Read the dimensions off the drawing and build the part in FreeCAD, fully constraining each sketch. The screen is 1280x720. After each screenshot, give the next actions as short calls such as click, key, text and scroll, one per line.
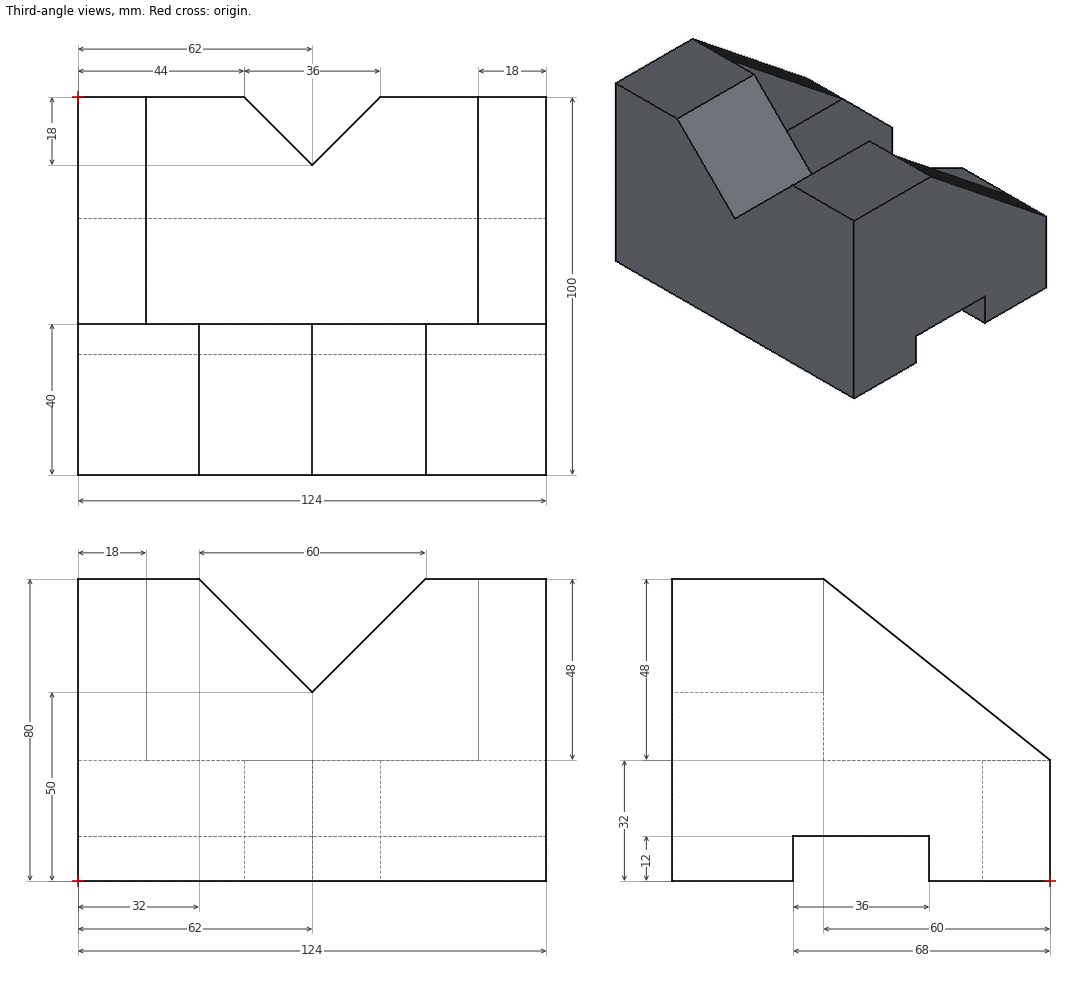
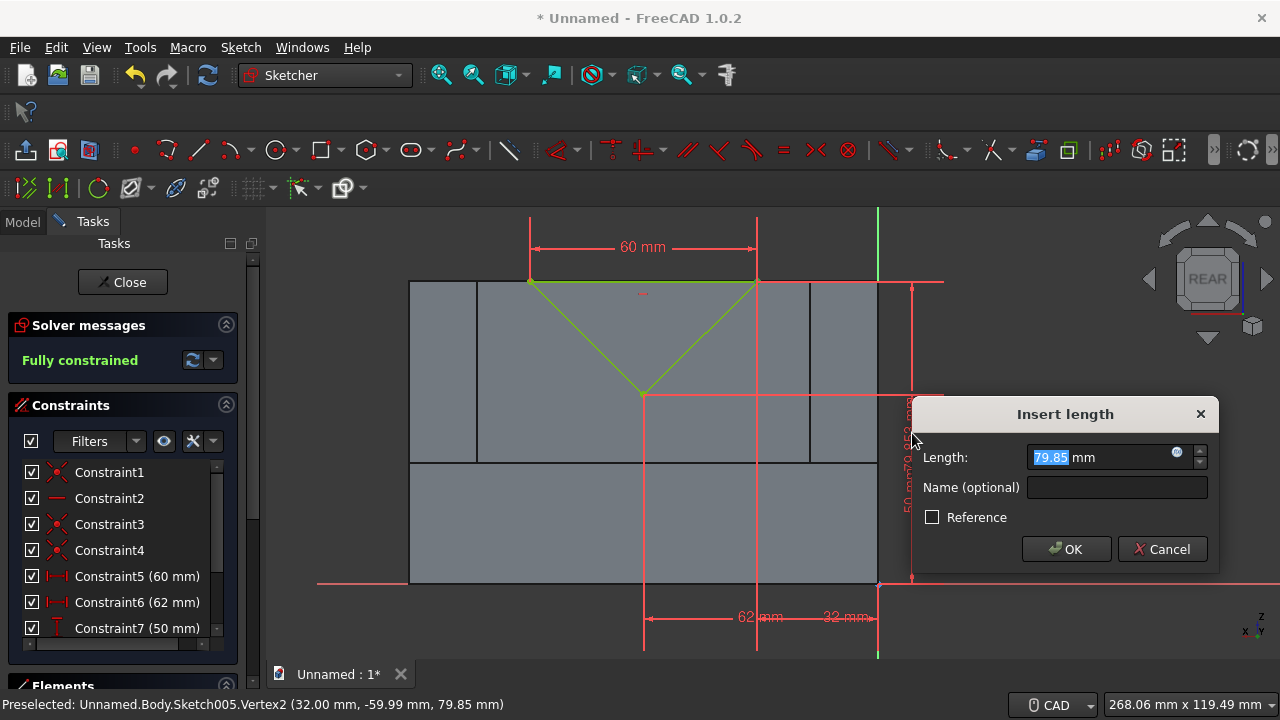
text(80)
key(Return)
key(Escape)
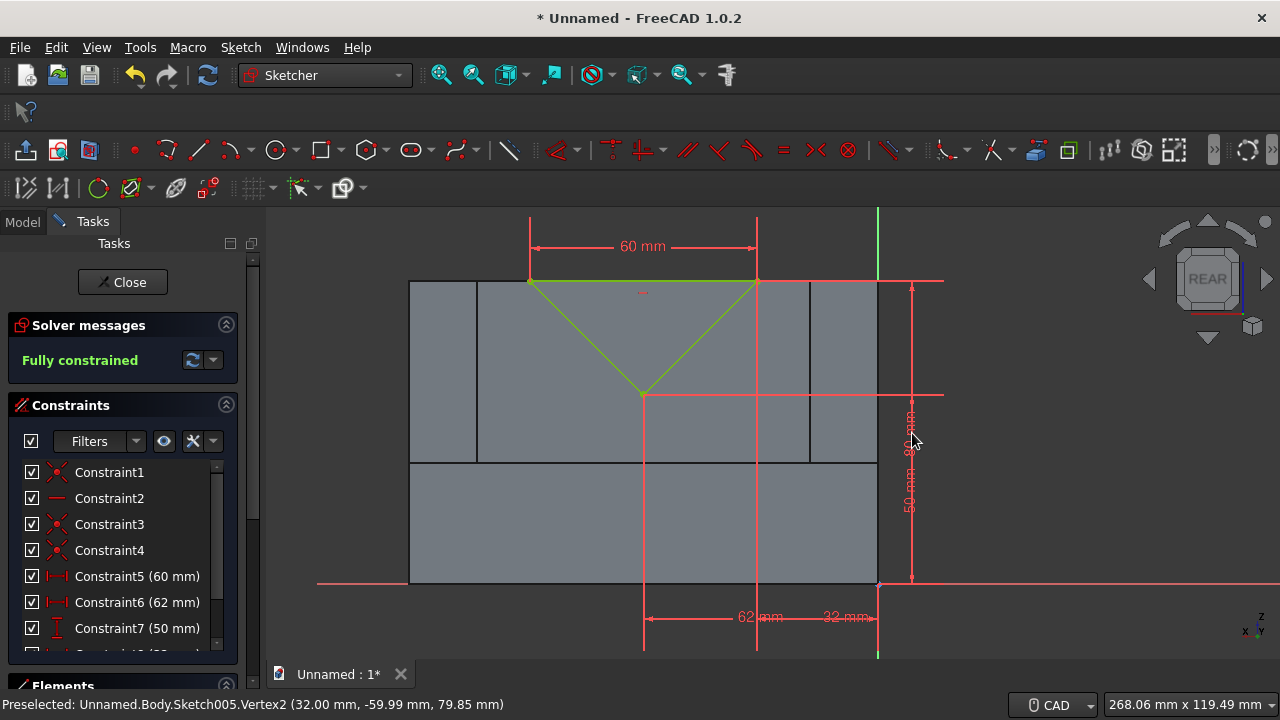
click(123, 282)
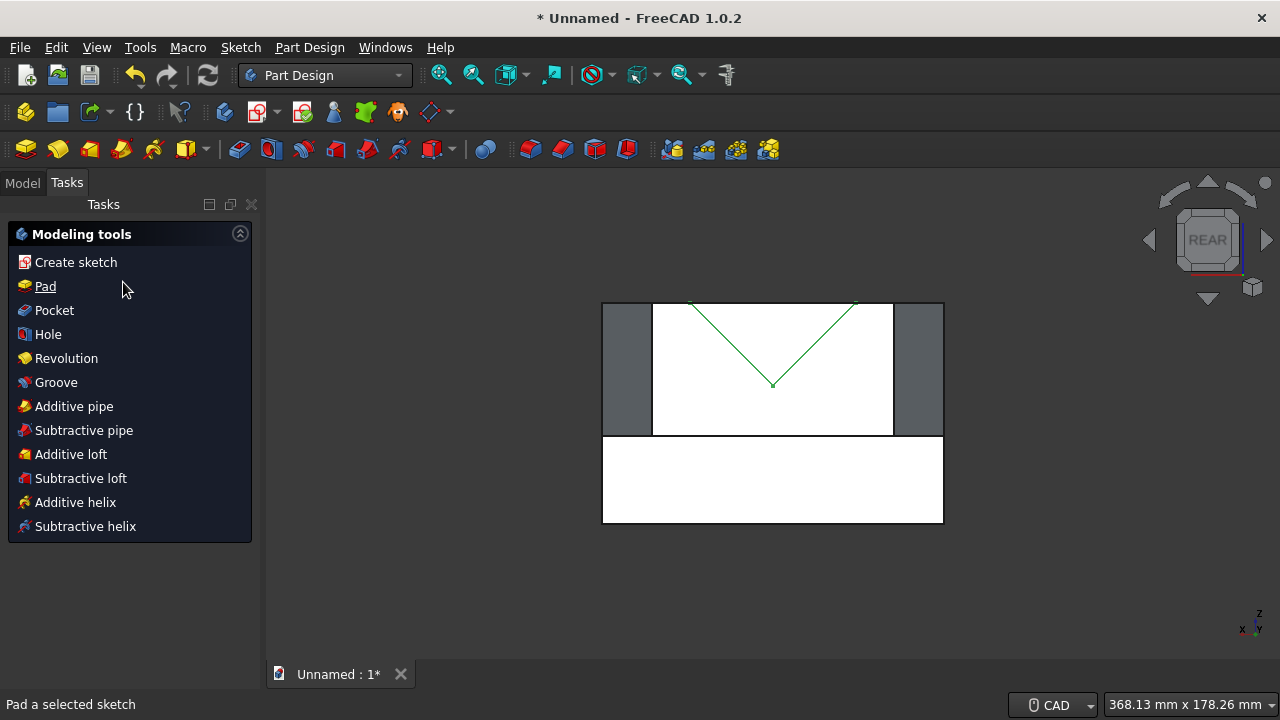
click(240, 150)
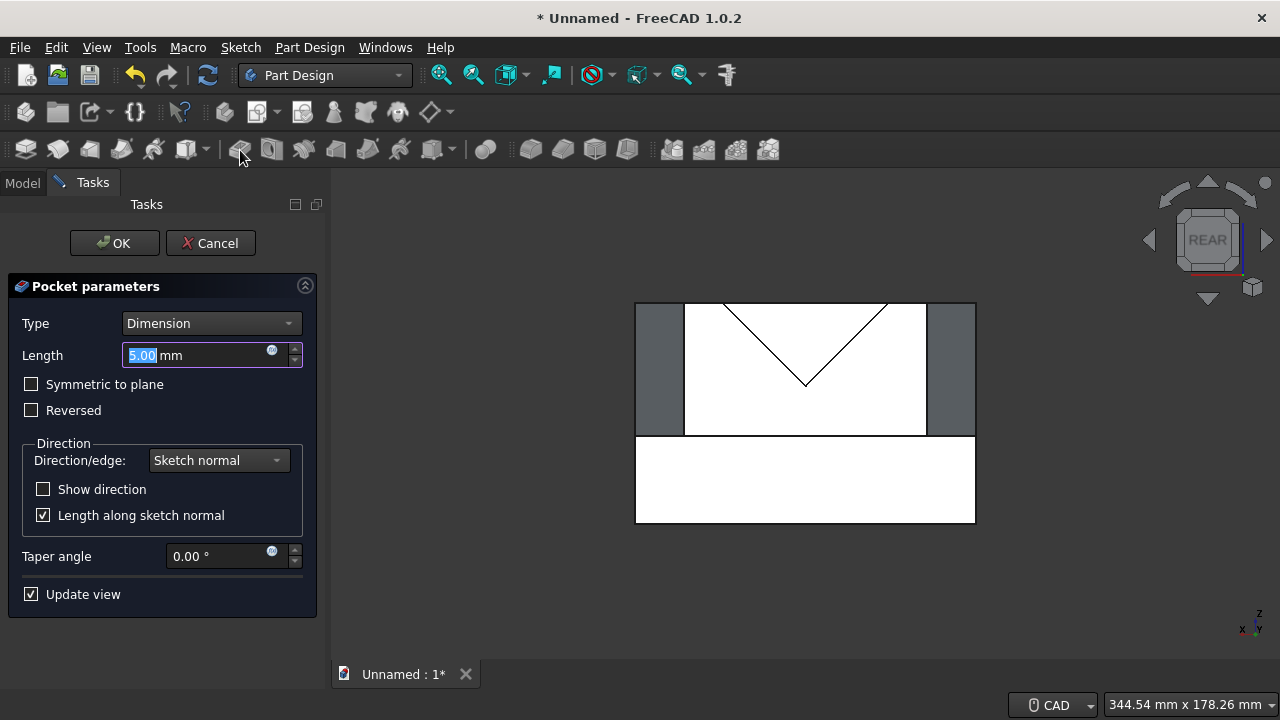
text(40)
key(Tab)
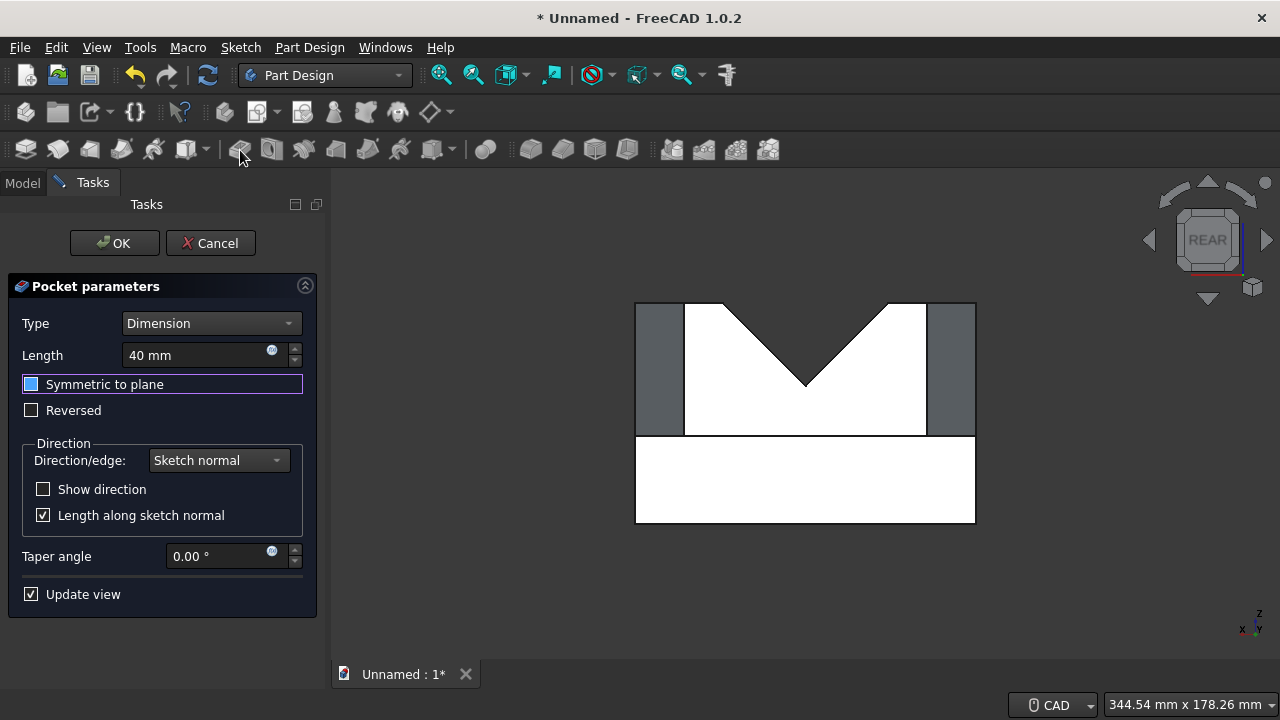
click(115, 243)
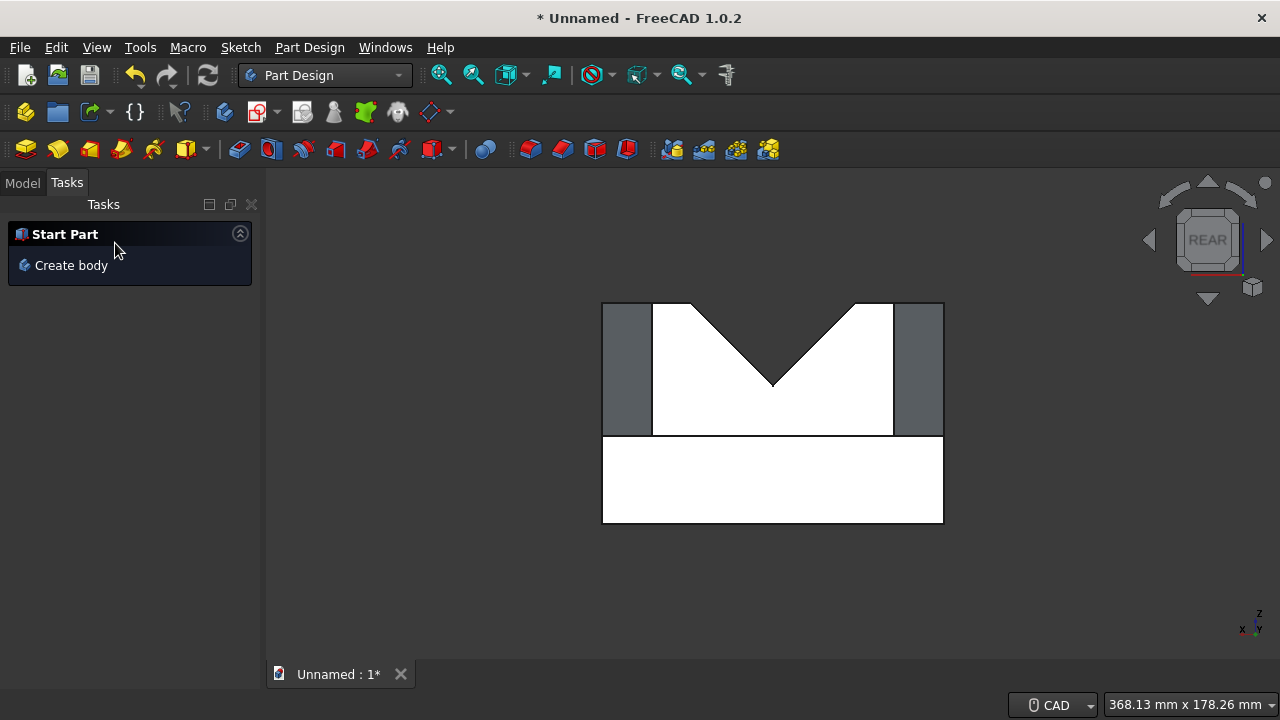
key(0)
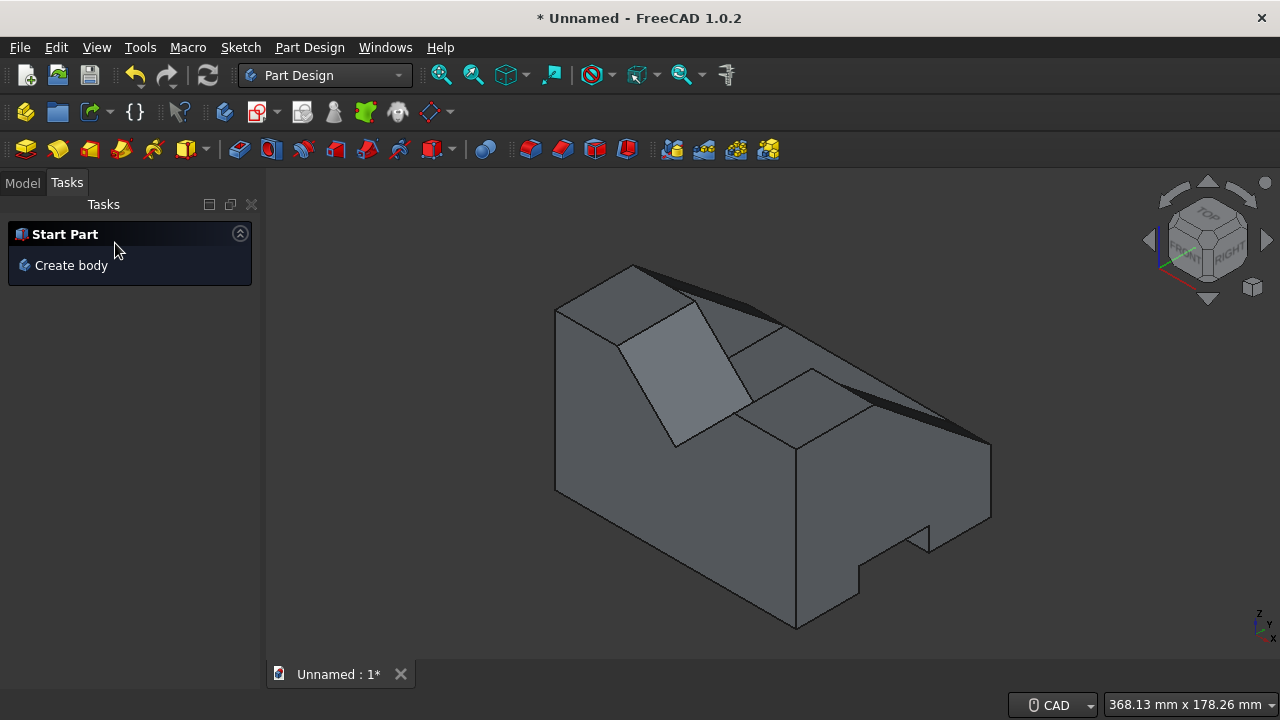
key(2)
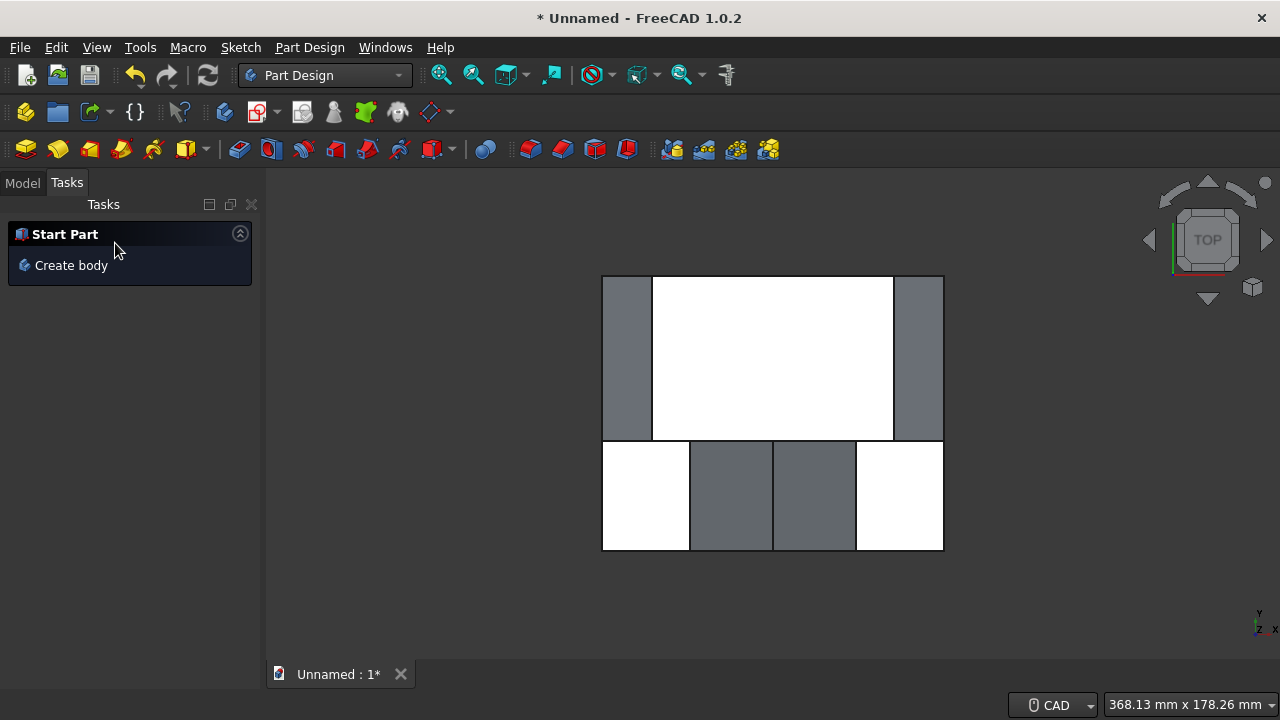
click(808, 357)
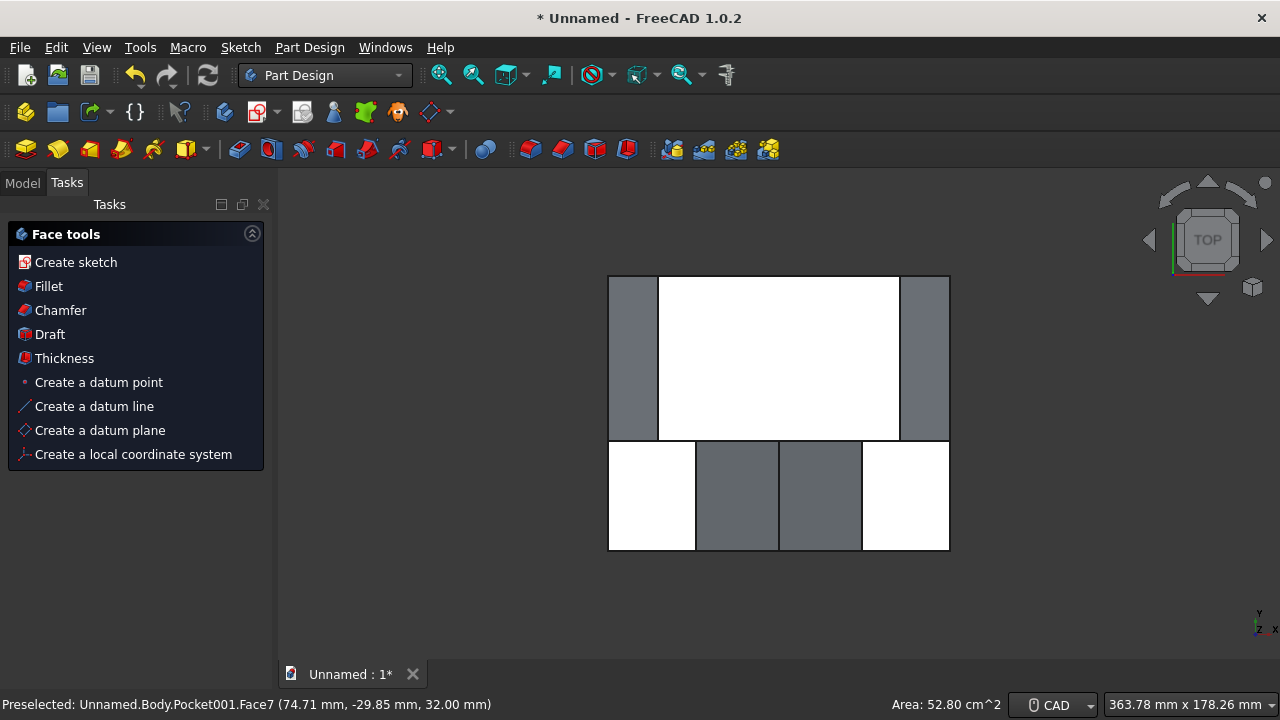
click(258, 112)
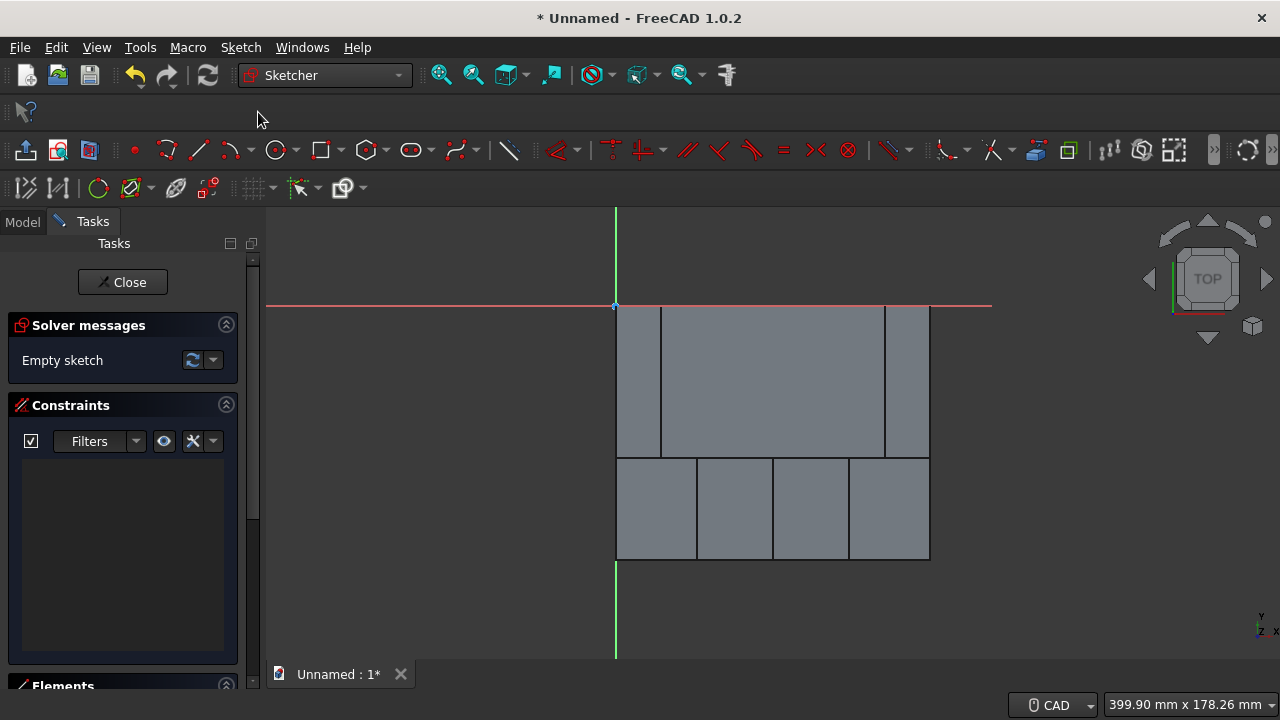
click(90, 150)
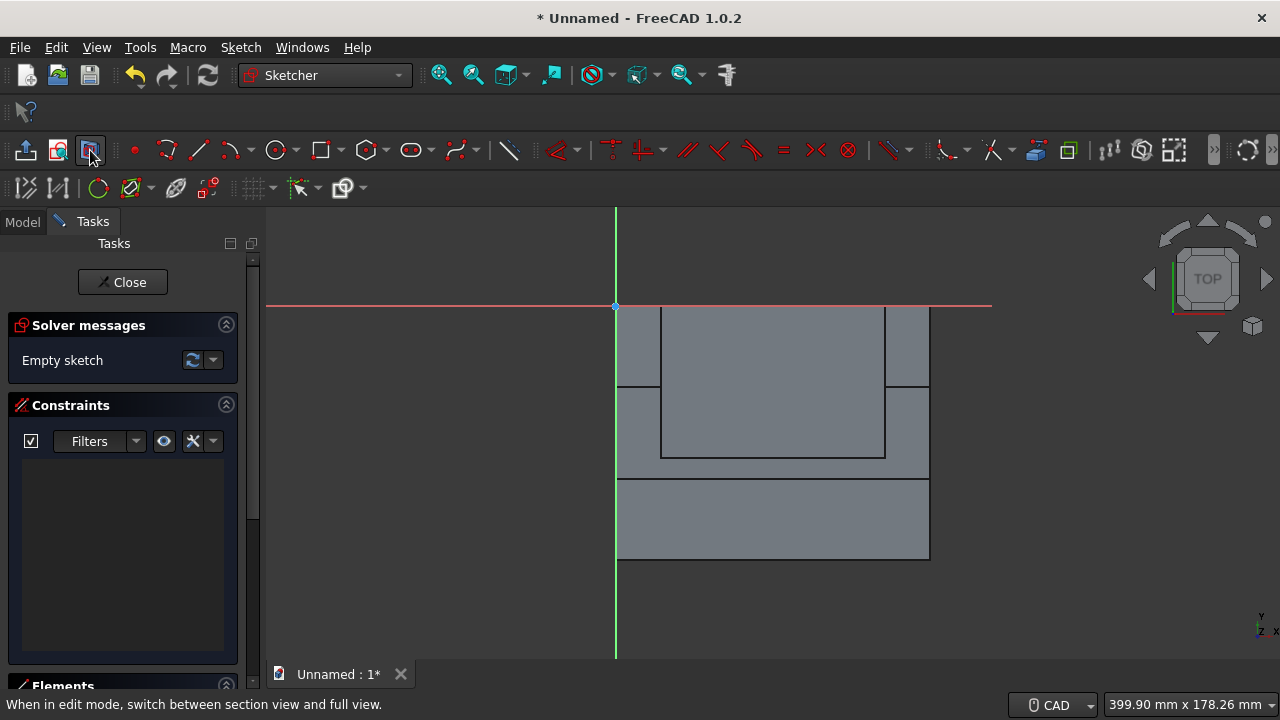
scroll(725, 269, up, 5)